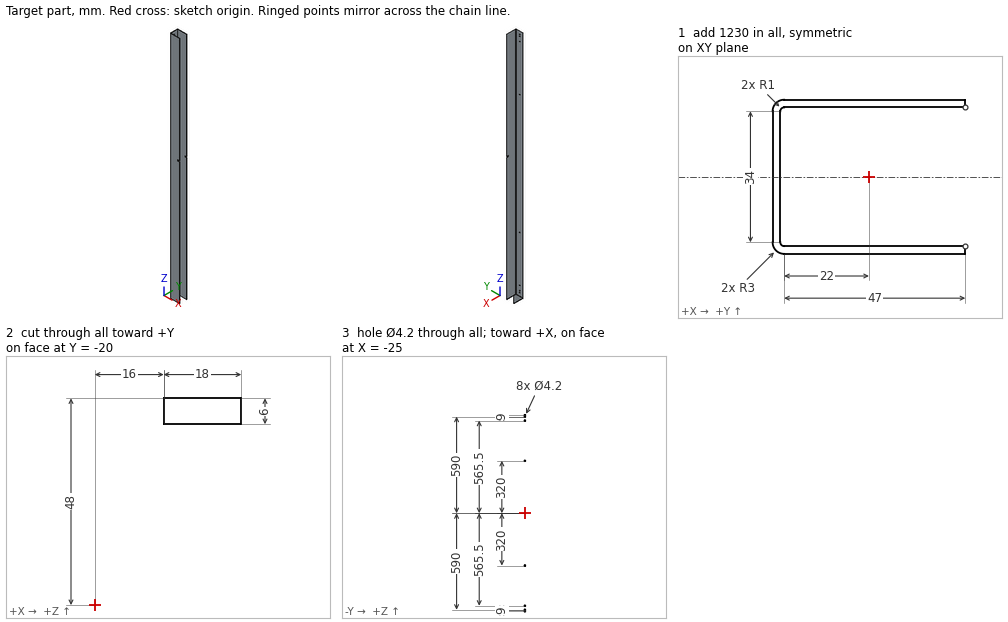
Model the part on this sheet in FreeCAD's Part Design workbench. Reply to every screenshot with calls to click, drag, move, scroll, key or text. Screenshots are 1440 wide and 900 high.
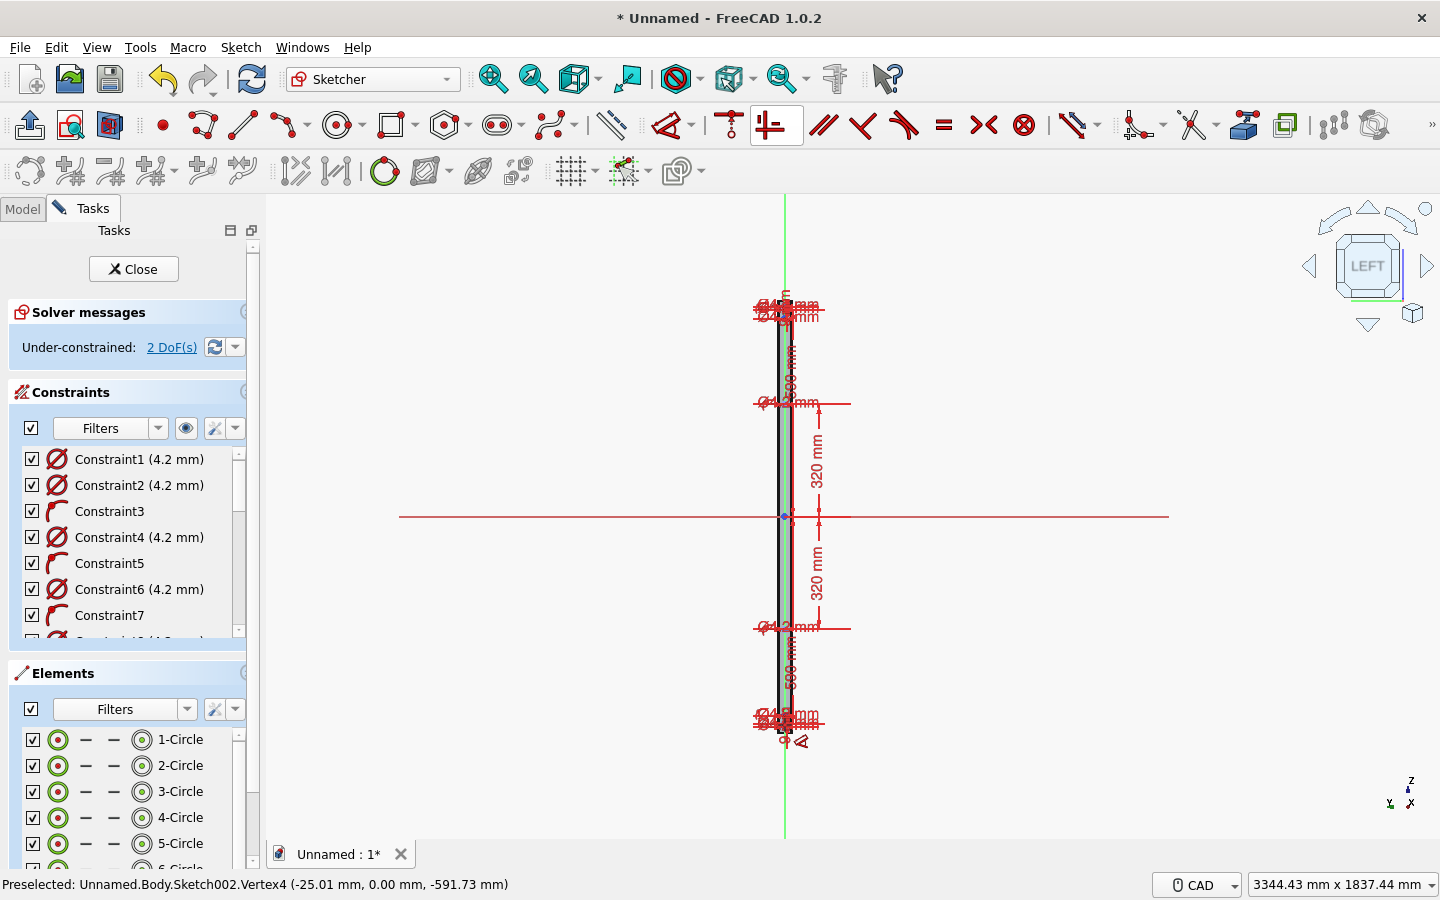
scroll(785, 319, up, 2)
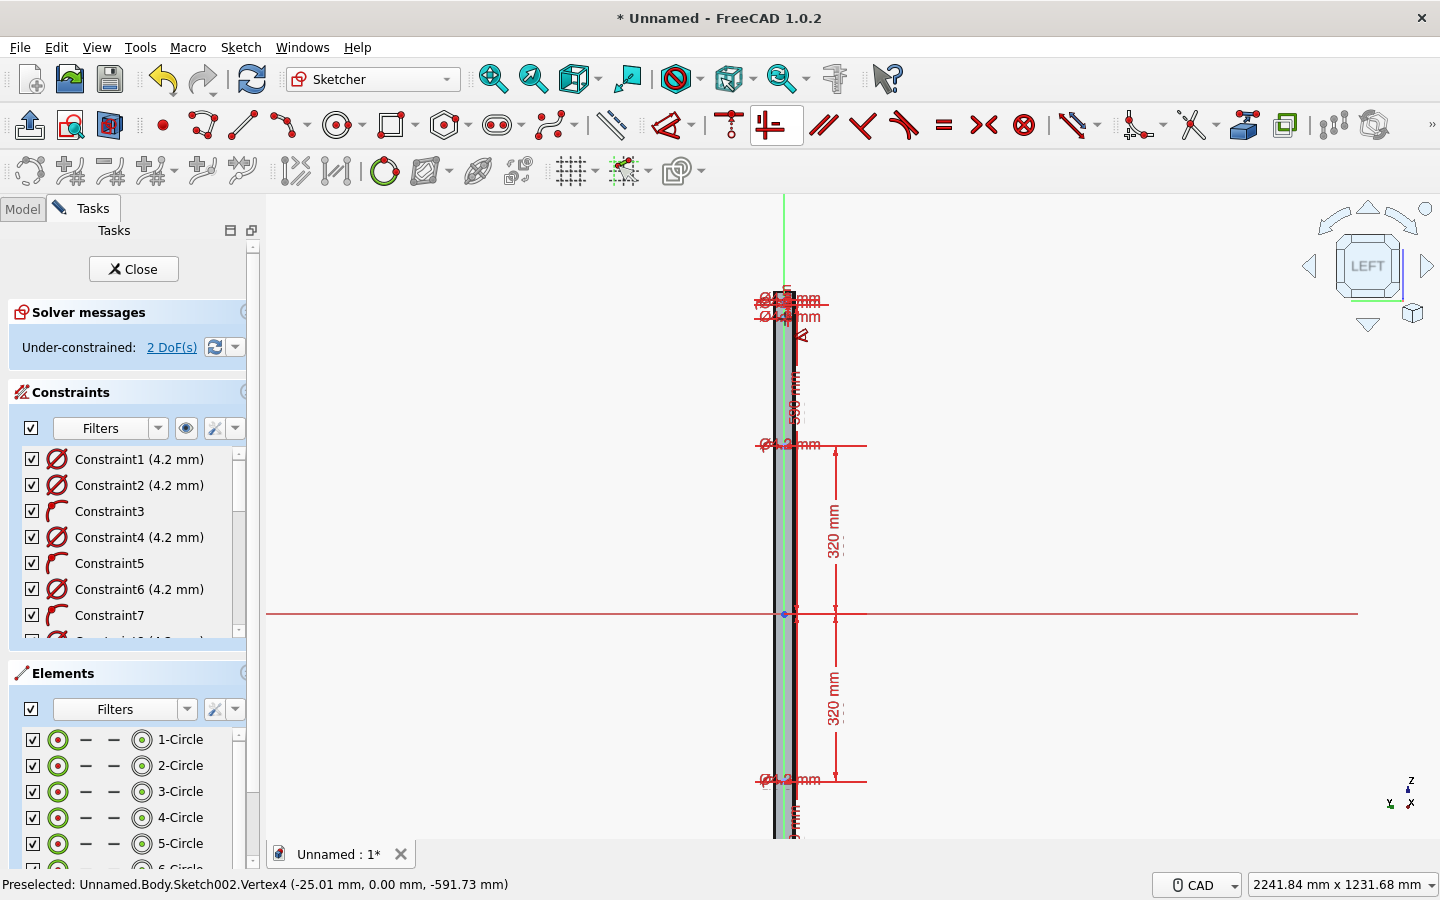
click(784, 319)
click(818, 466)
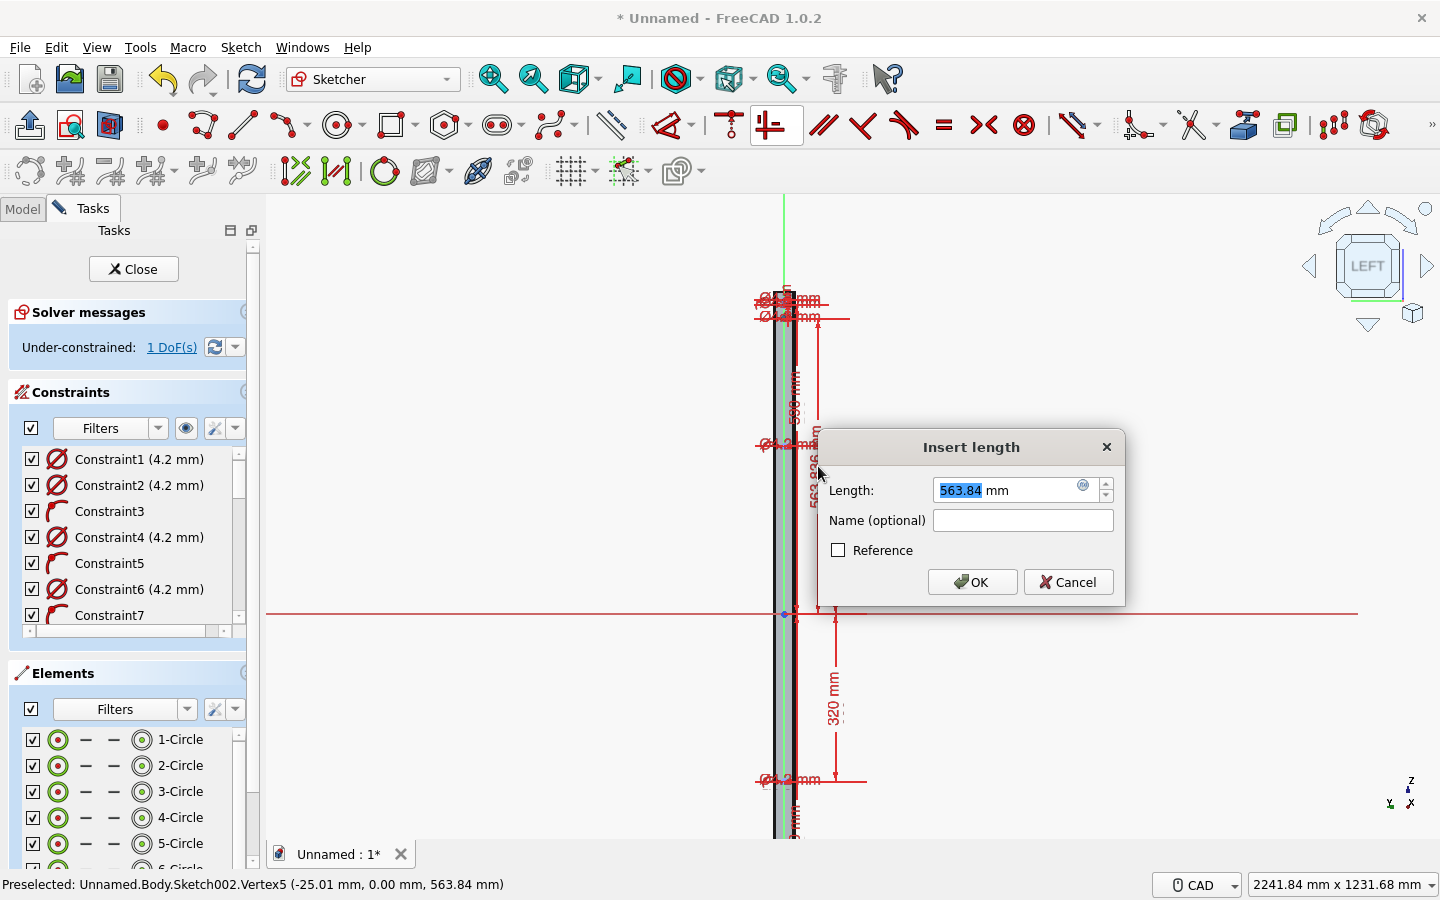
text(565.5)
key(Return)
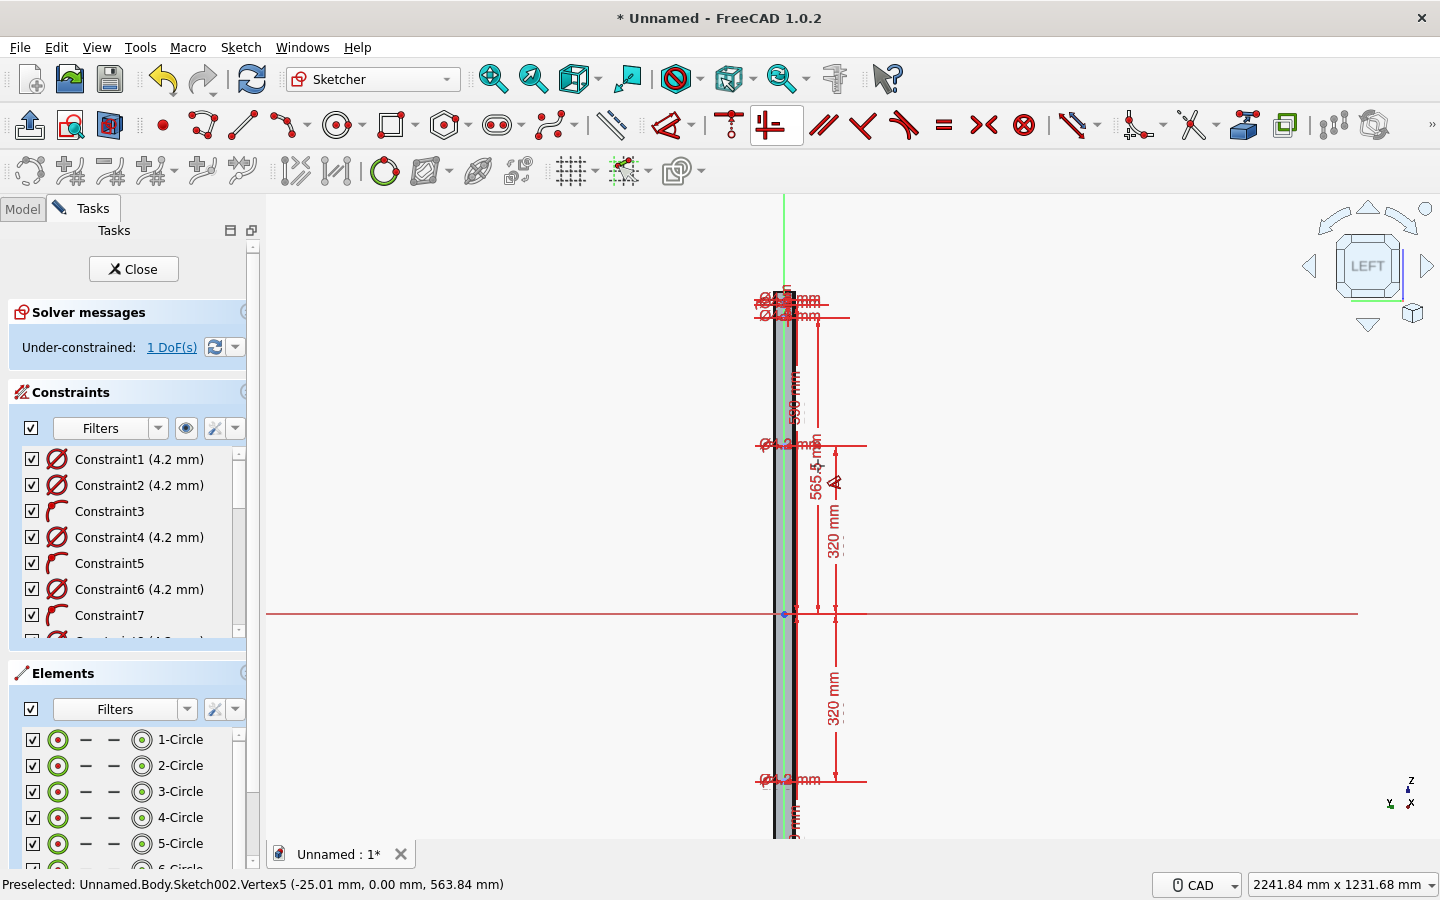
scroll(785, 318, down, 2)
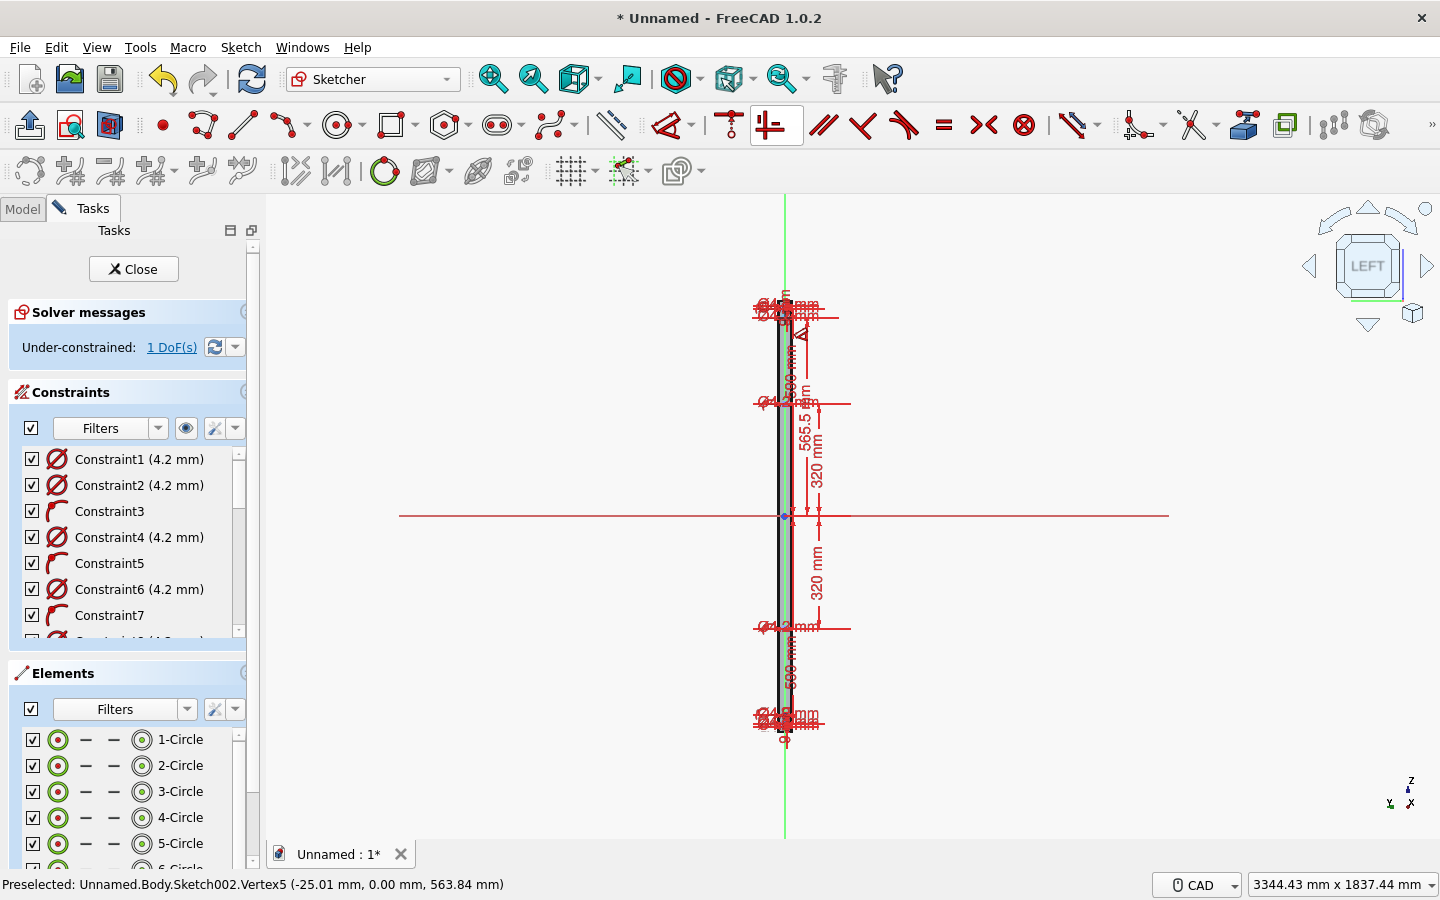
scroll(785, 715, up, 3)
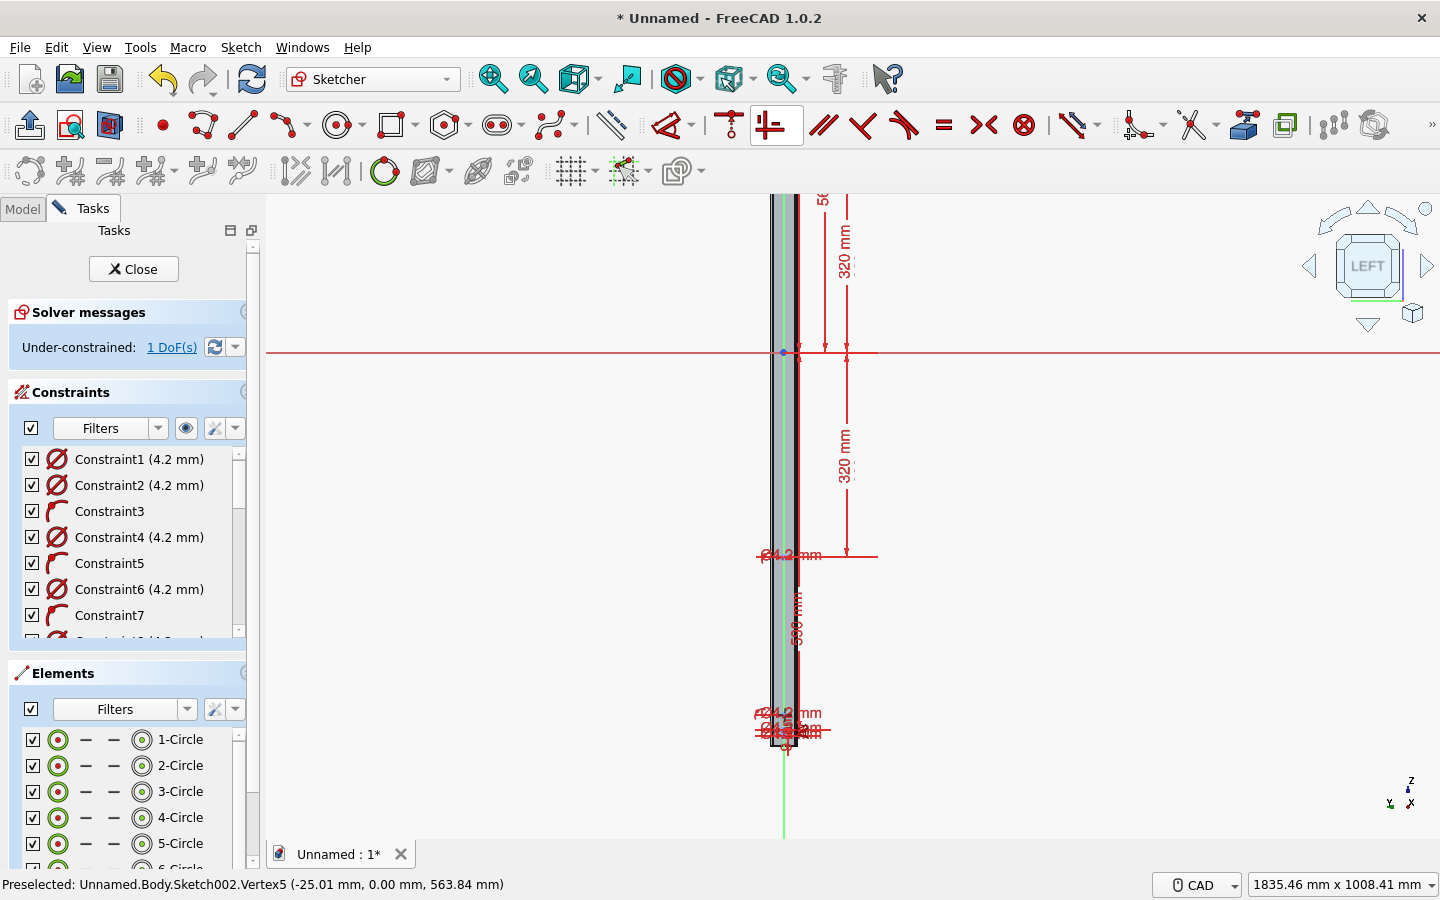
click(784, 715)
click(818, 534)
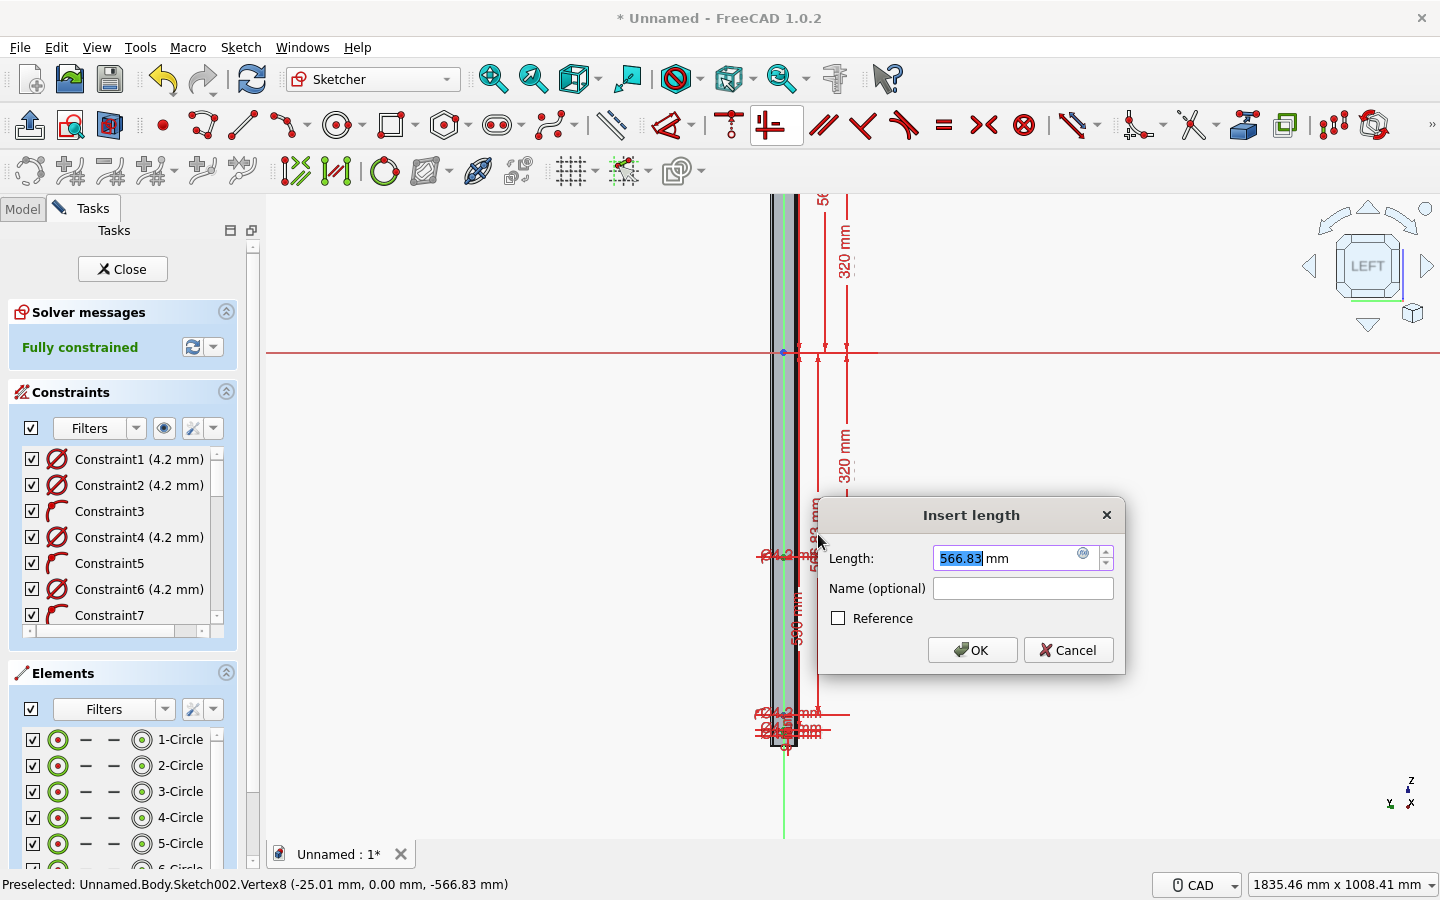
text(565.5)
key(Return)
key(Escape)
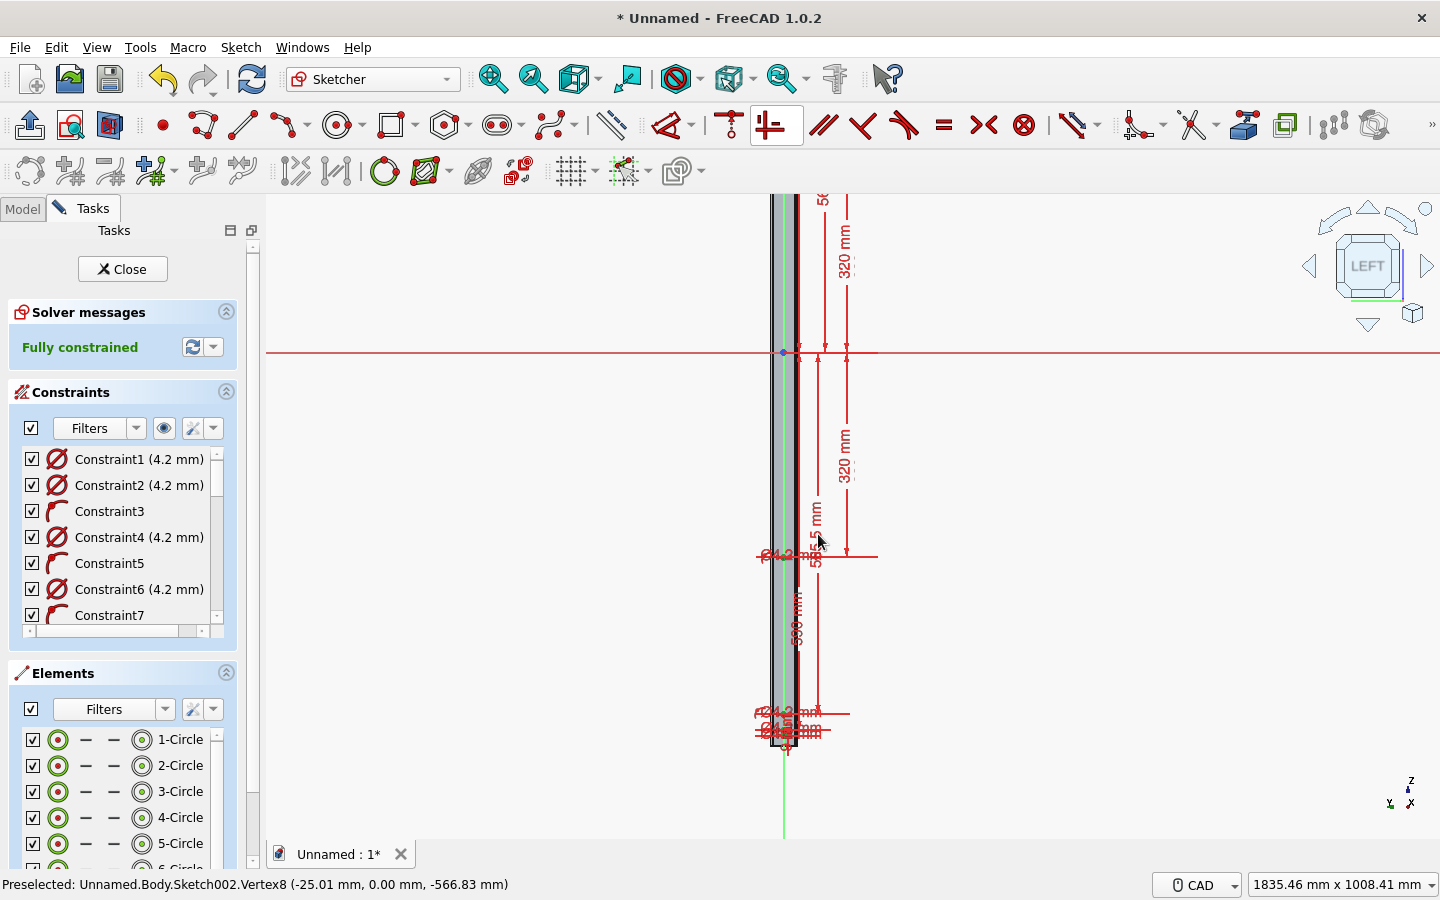
click(123, 269)